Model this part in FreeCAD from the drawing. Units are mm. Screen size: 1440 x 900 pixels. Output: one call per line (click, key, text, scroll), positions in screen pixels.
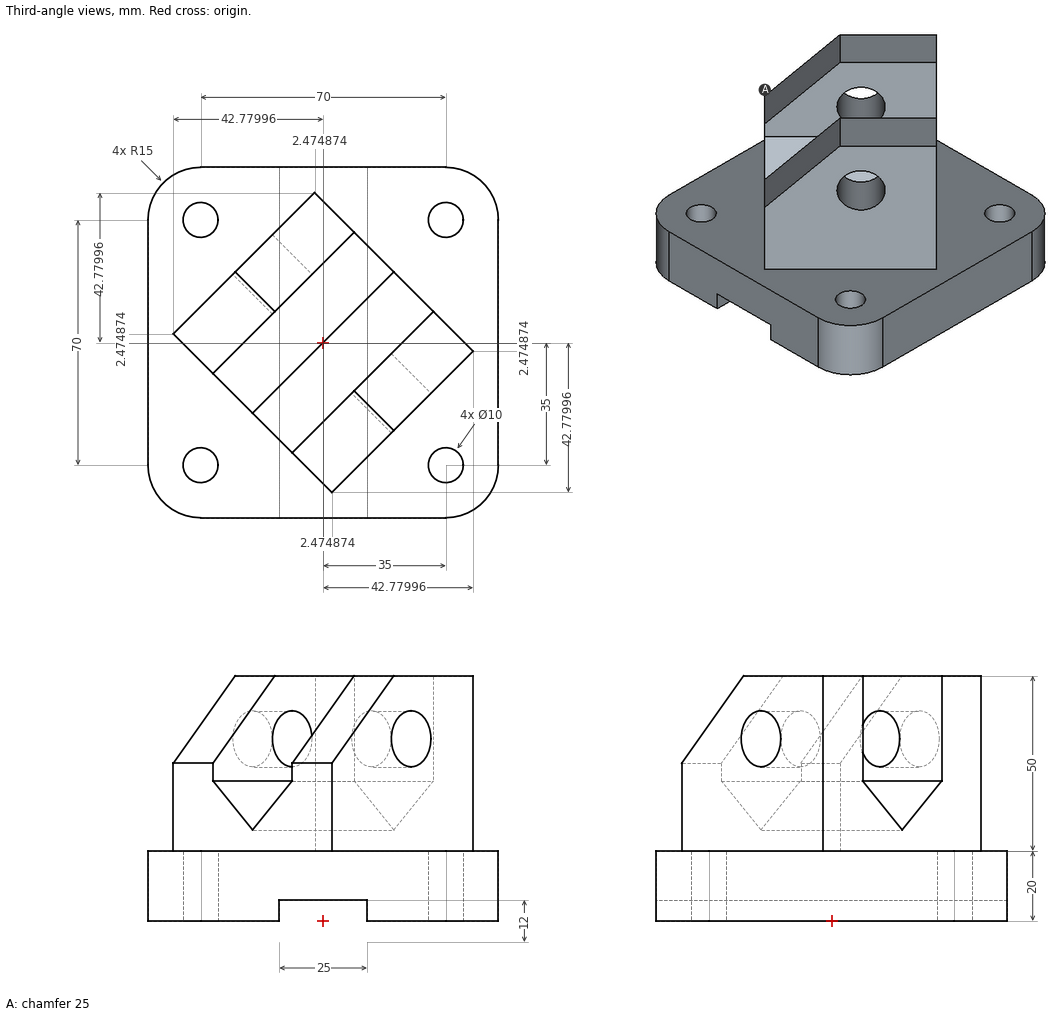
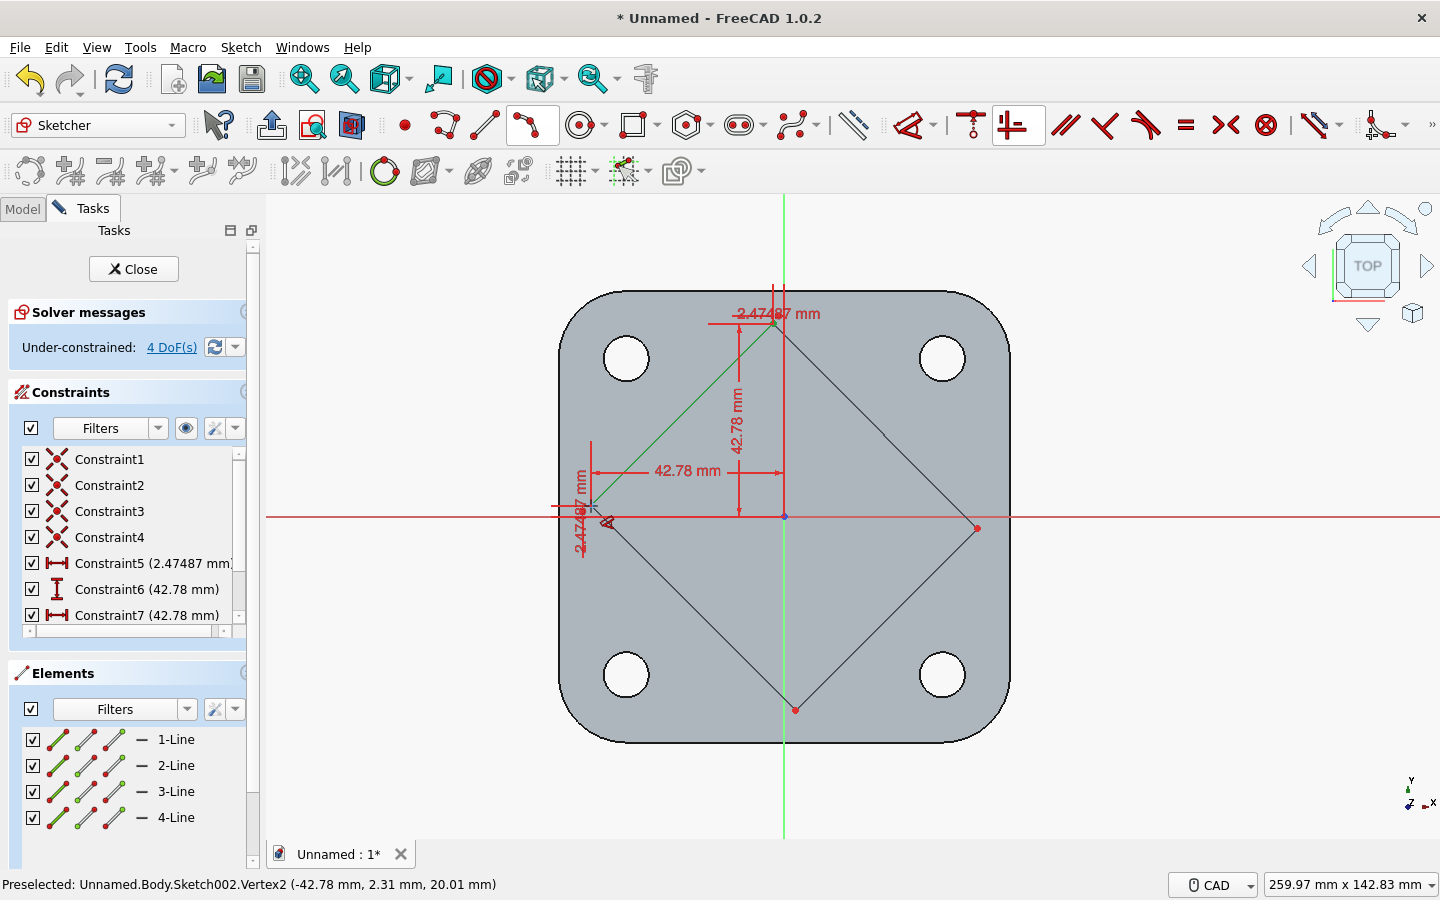
scroll(796, 711, up, 7)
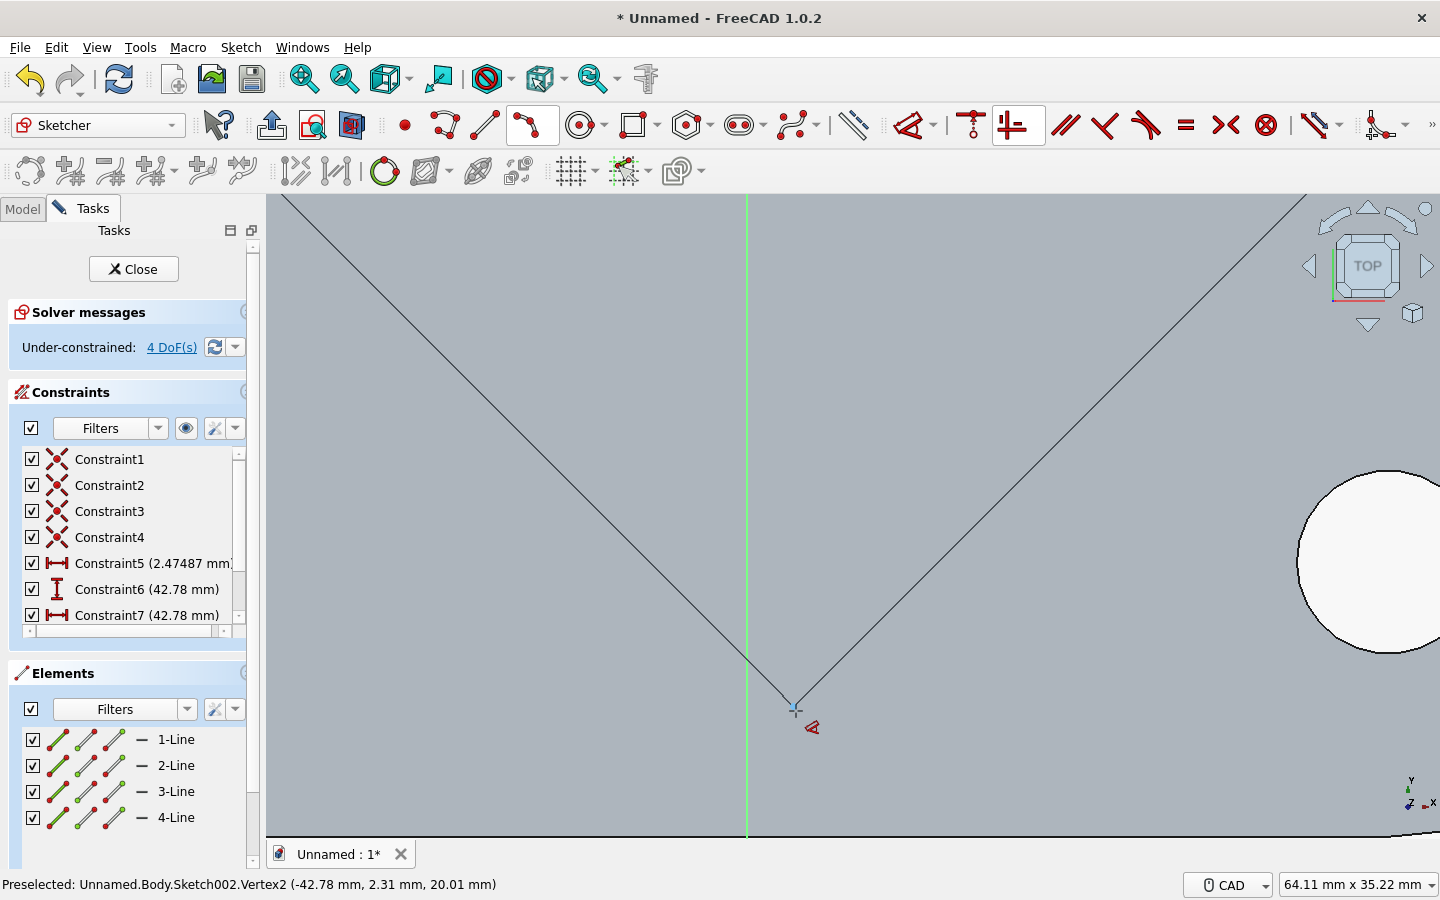
click(794, 707)
click(771, 741)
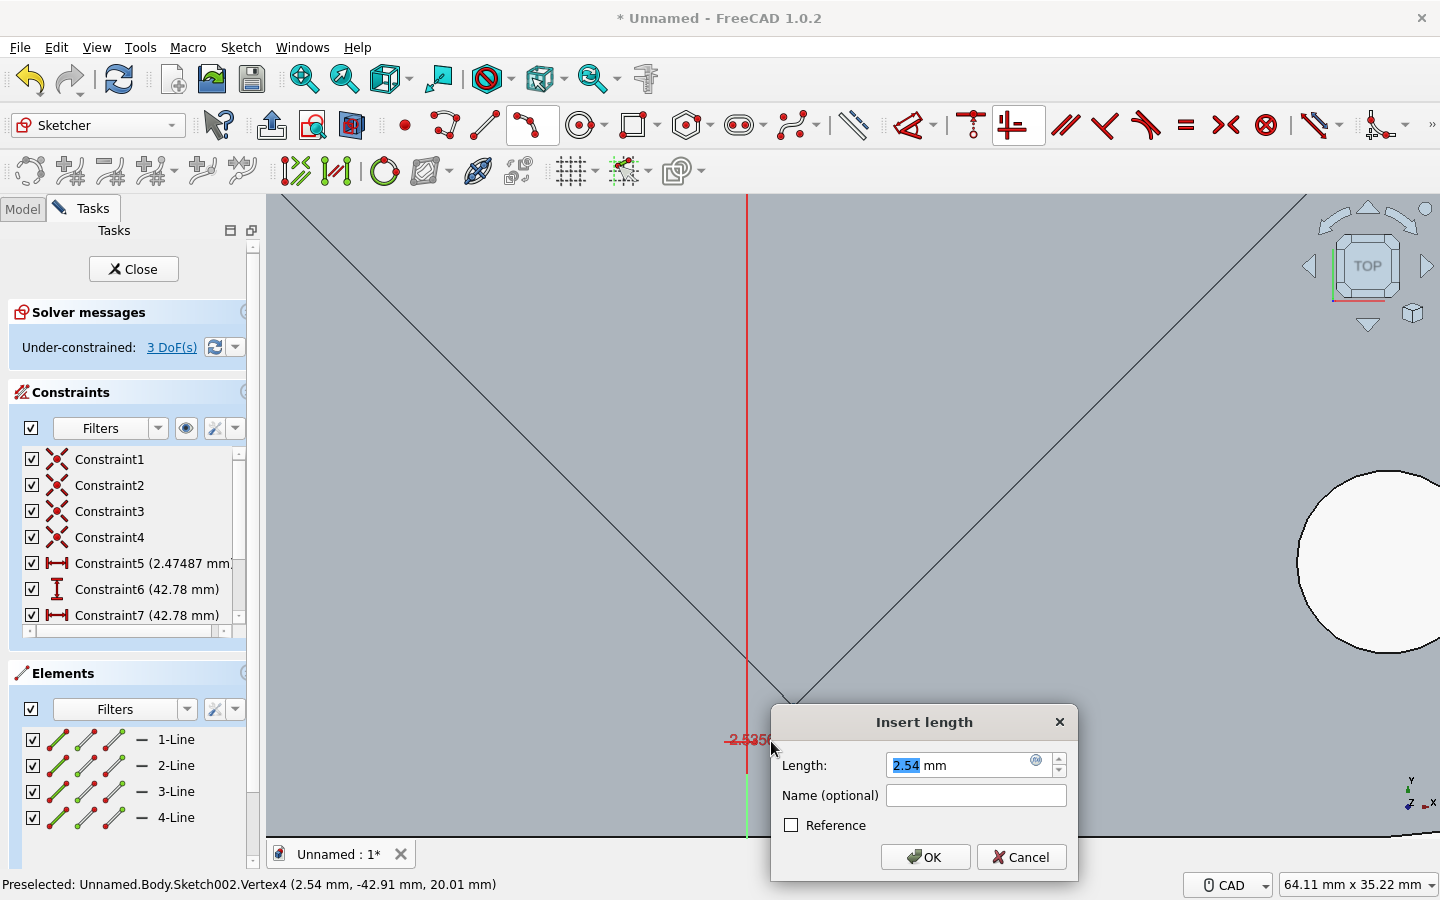
text(2.474874)
key(Return)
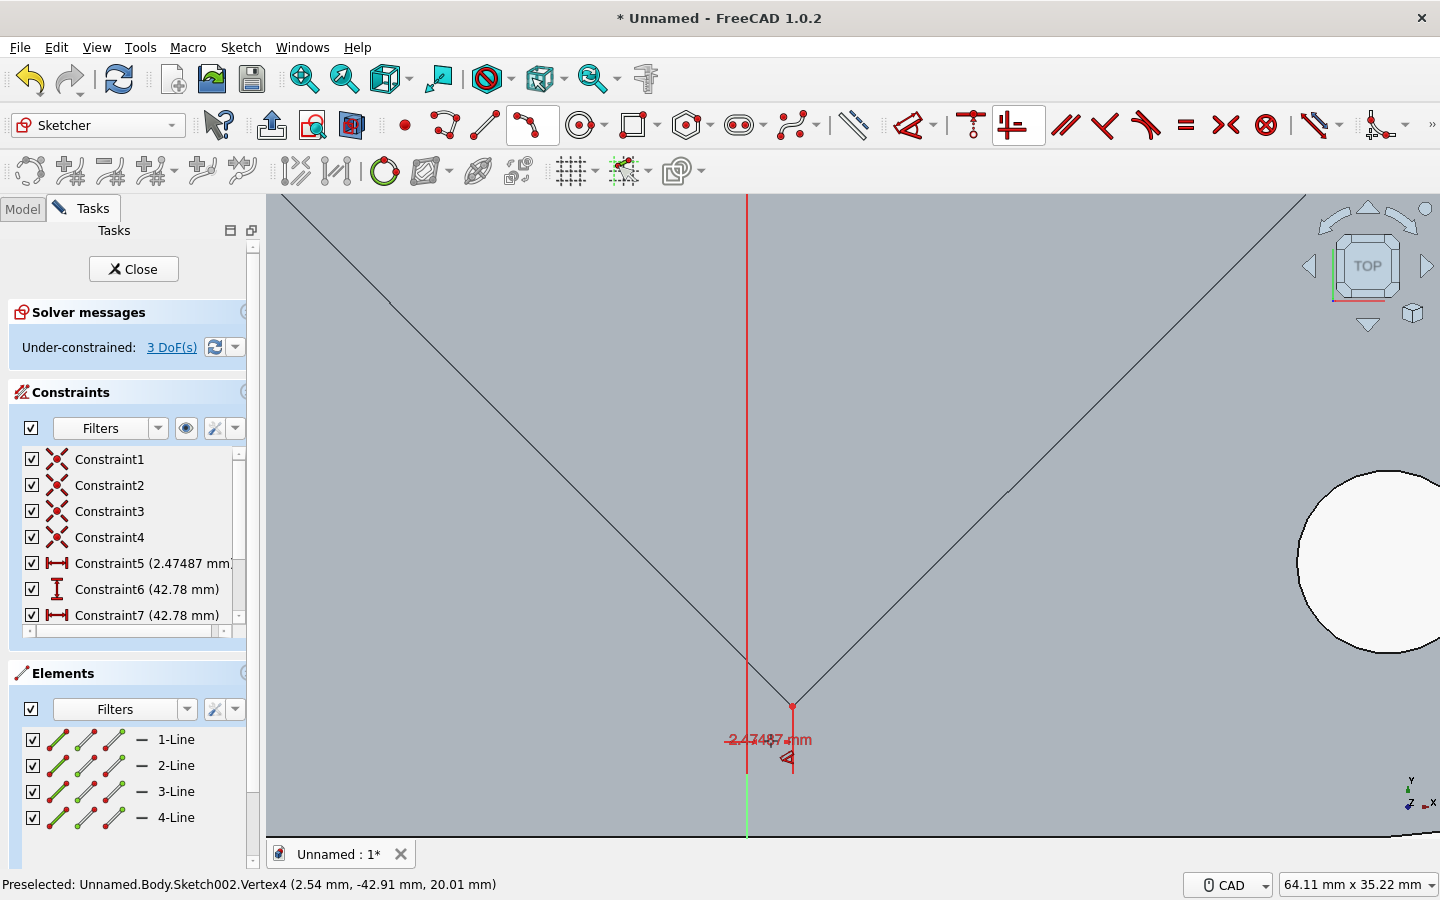
scroll(797, 711, down, 7)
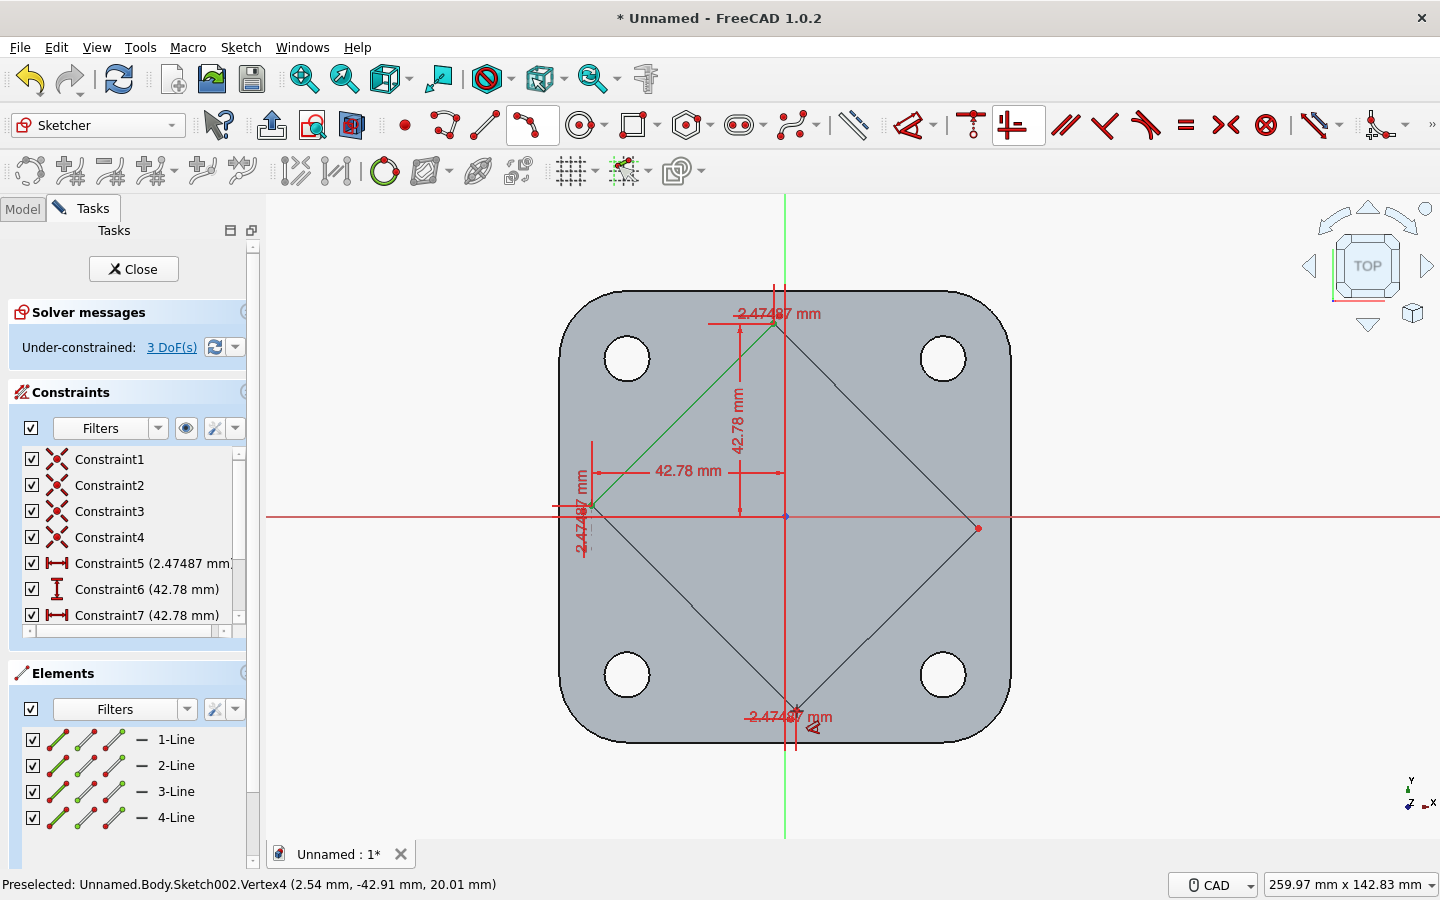
click(796, 711)
click(830, 614)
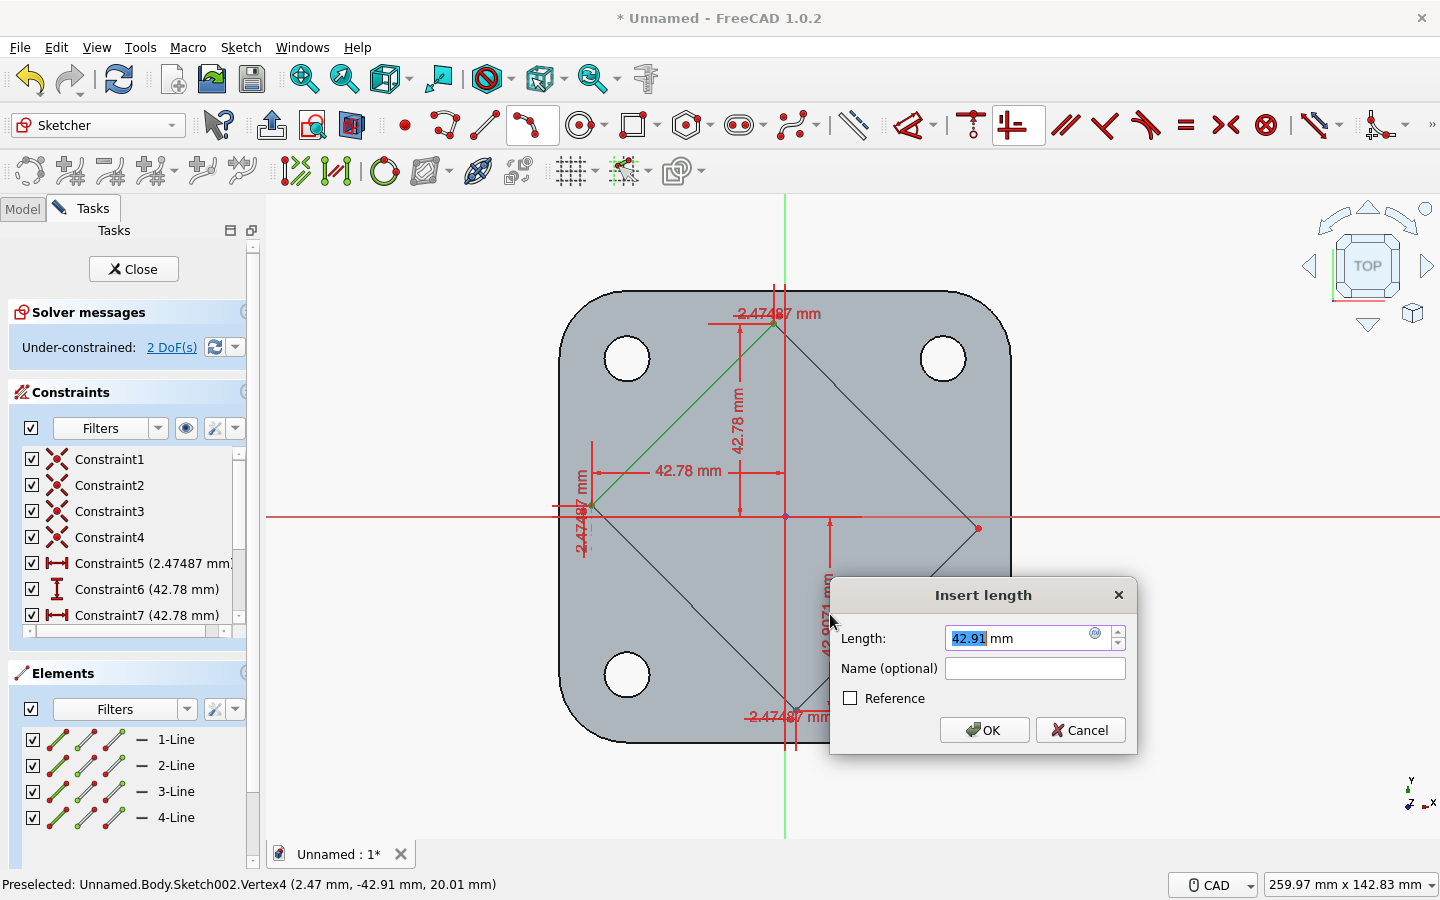
text(42.77996)
key(Return)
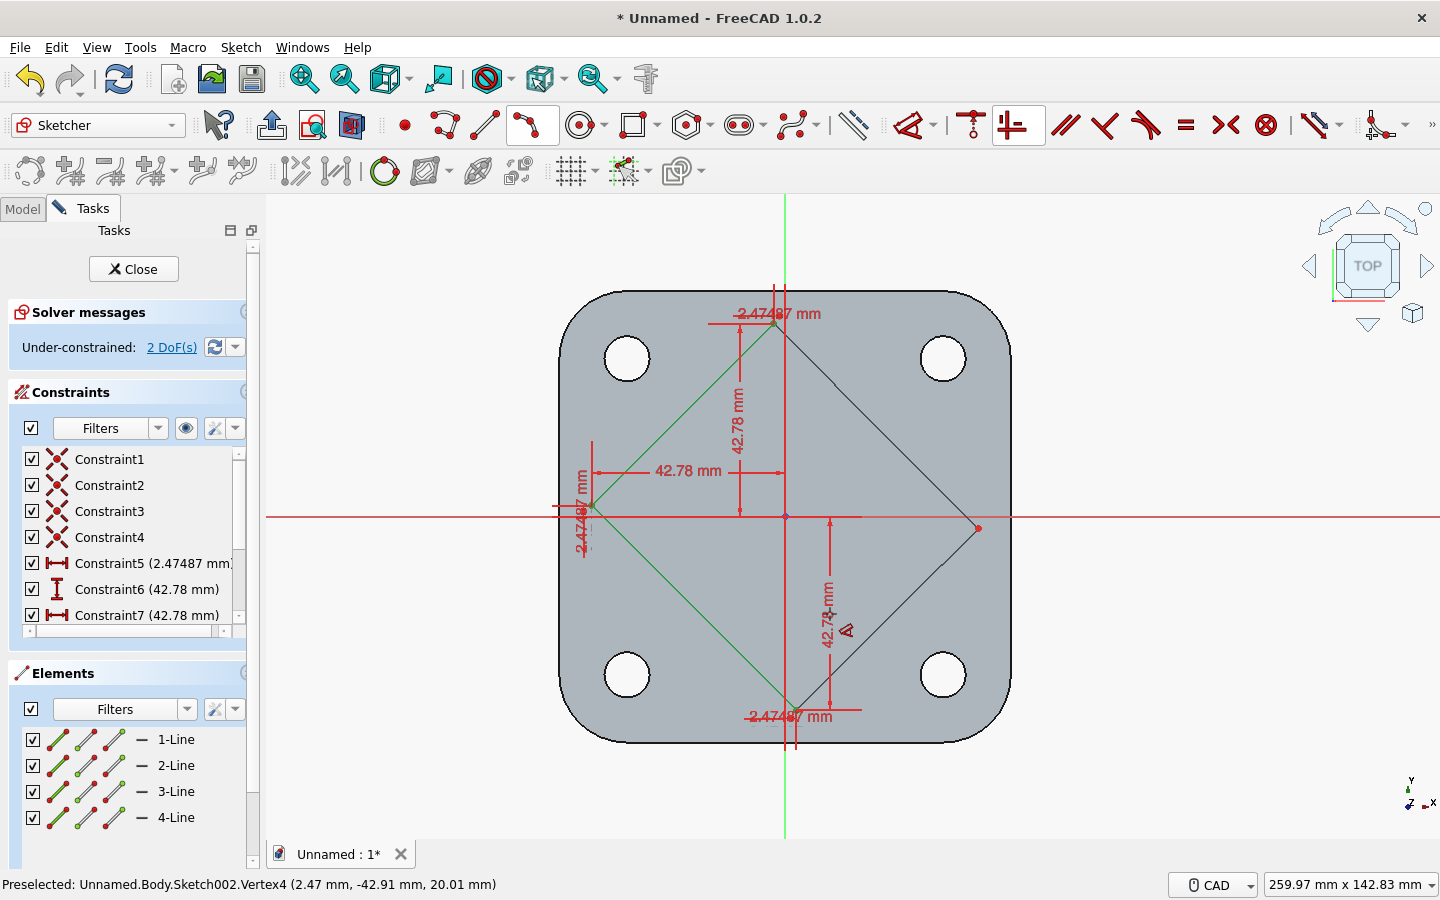
click(978, 529)
click(882, 563)